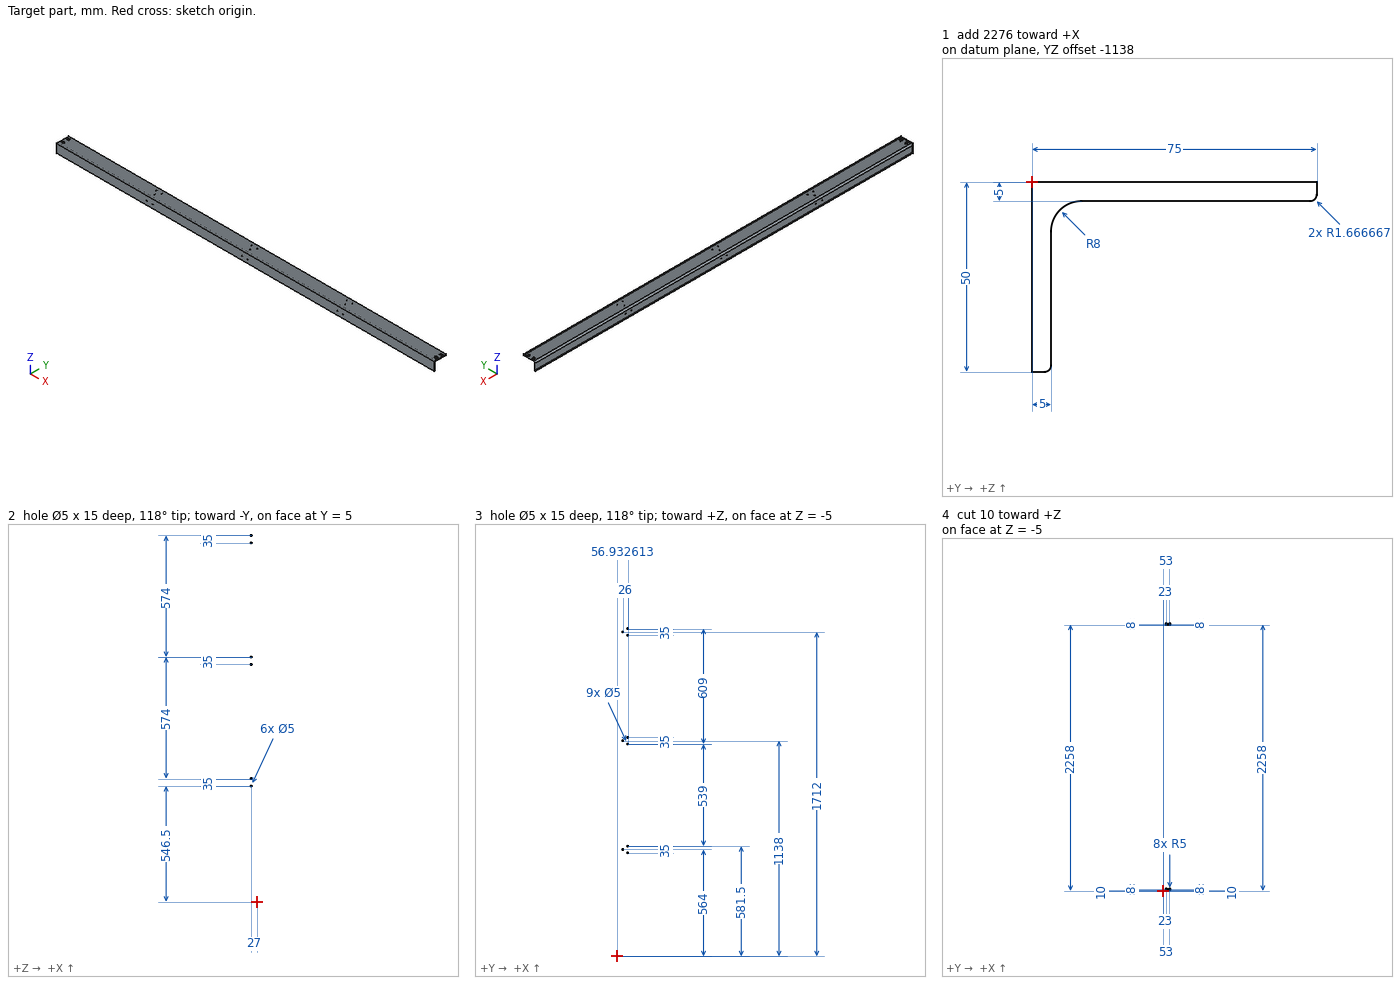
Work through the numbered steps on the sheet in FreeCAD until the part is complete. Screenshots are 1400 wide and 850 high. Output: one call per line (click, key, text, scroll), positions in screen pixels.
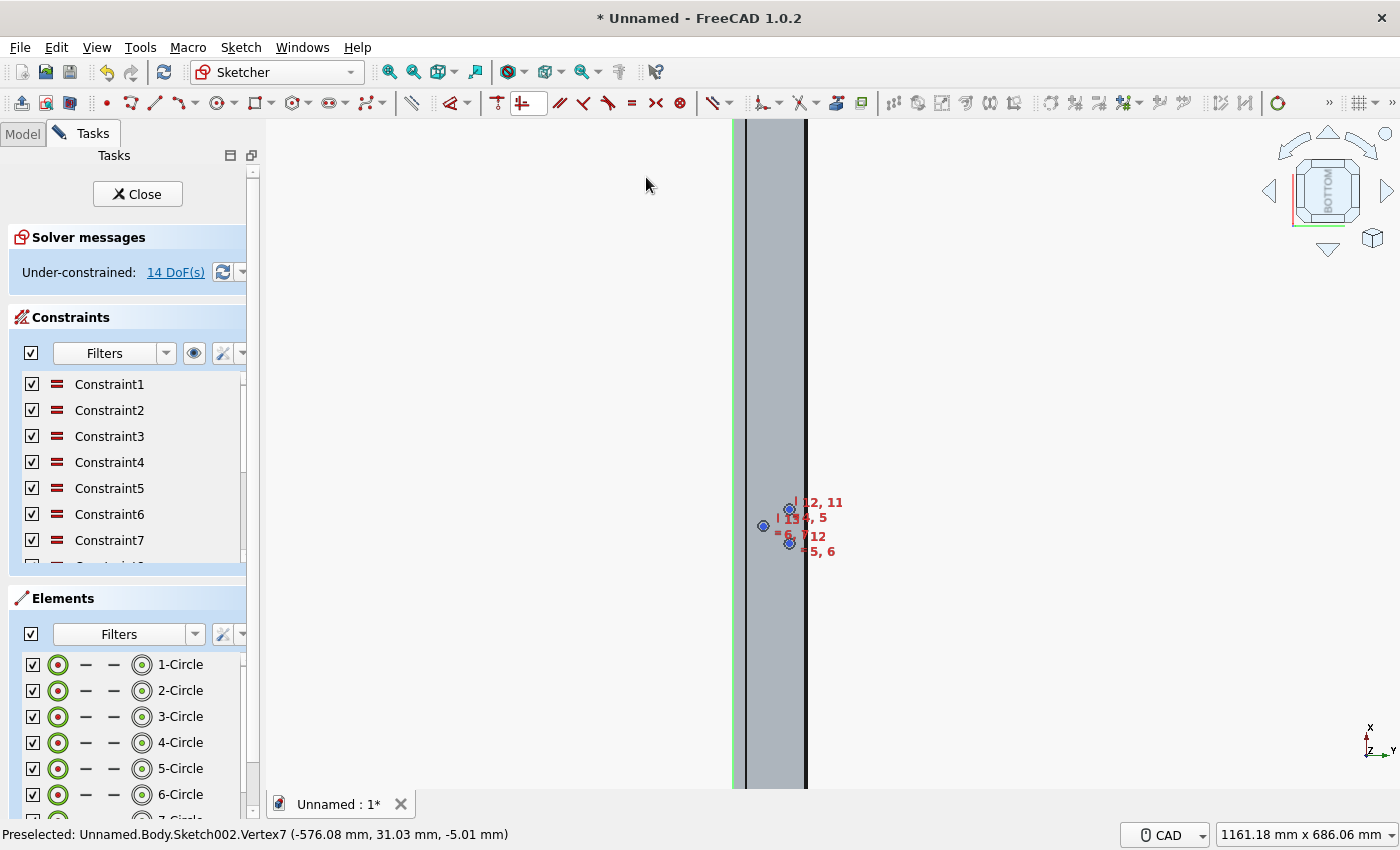
scroll(765, 528, down, 7)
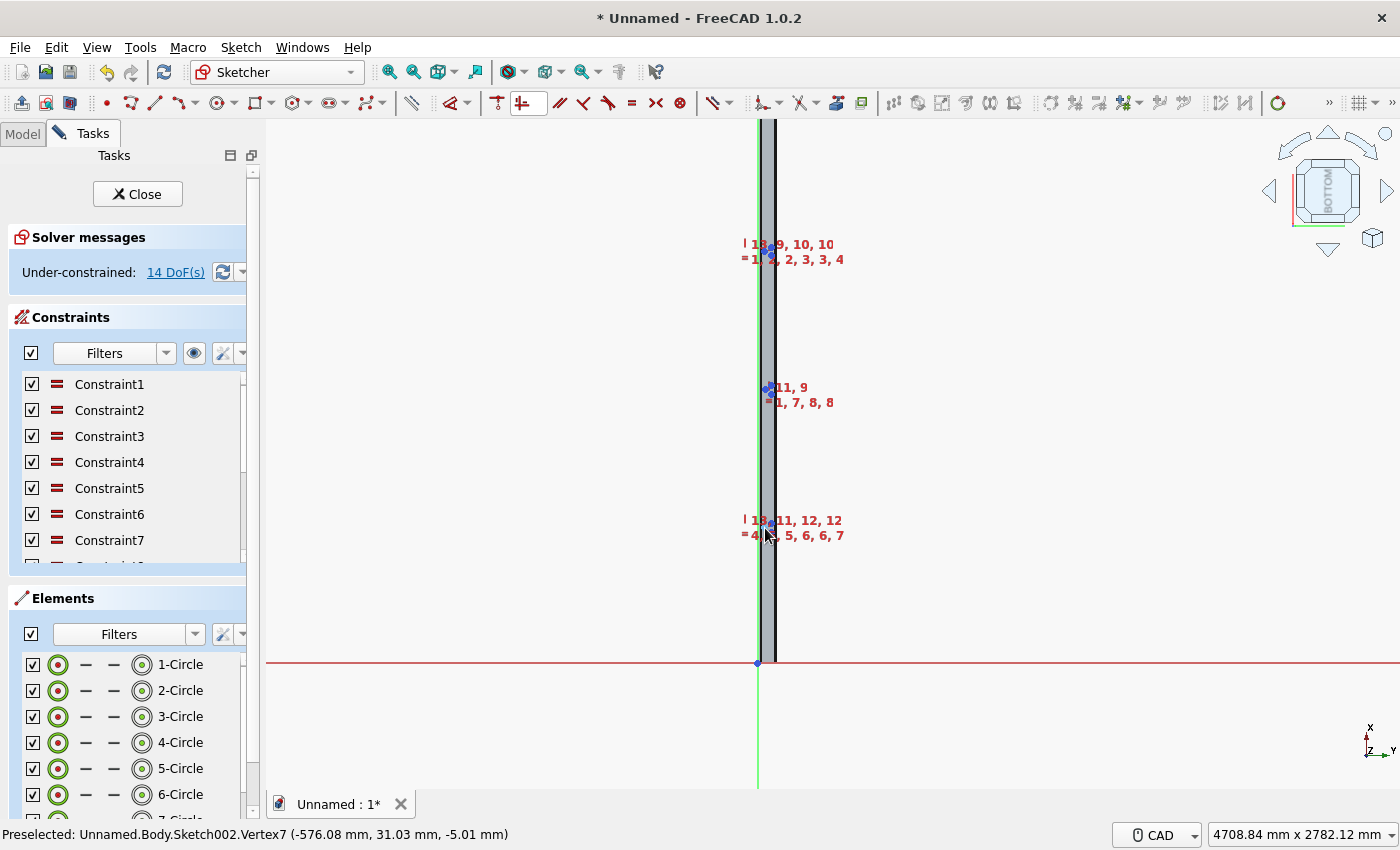
scroll(771, 394, up, 3)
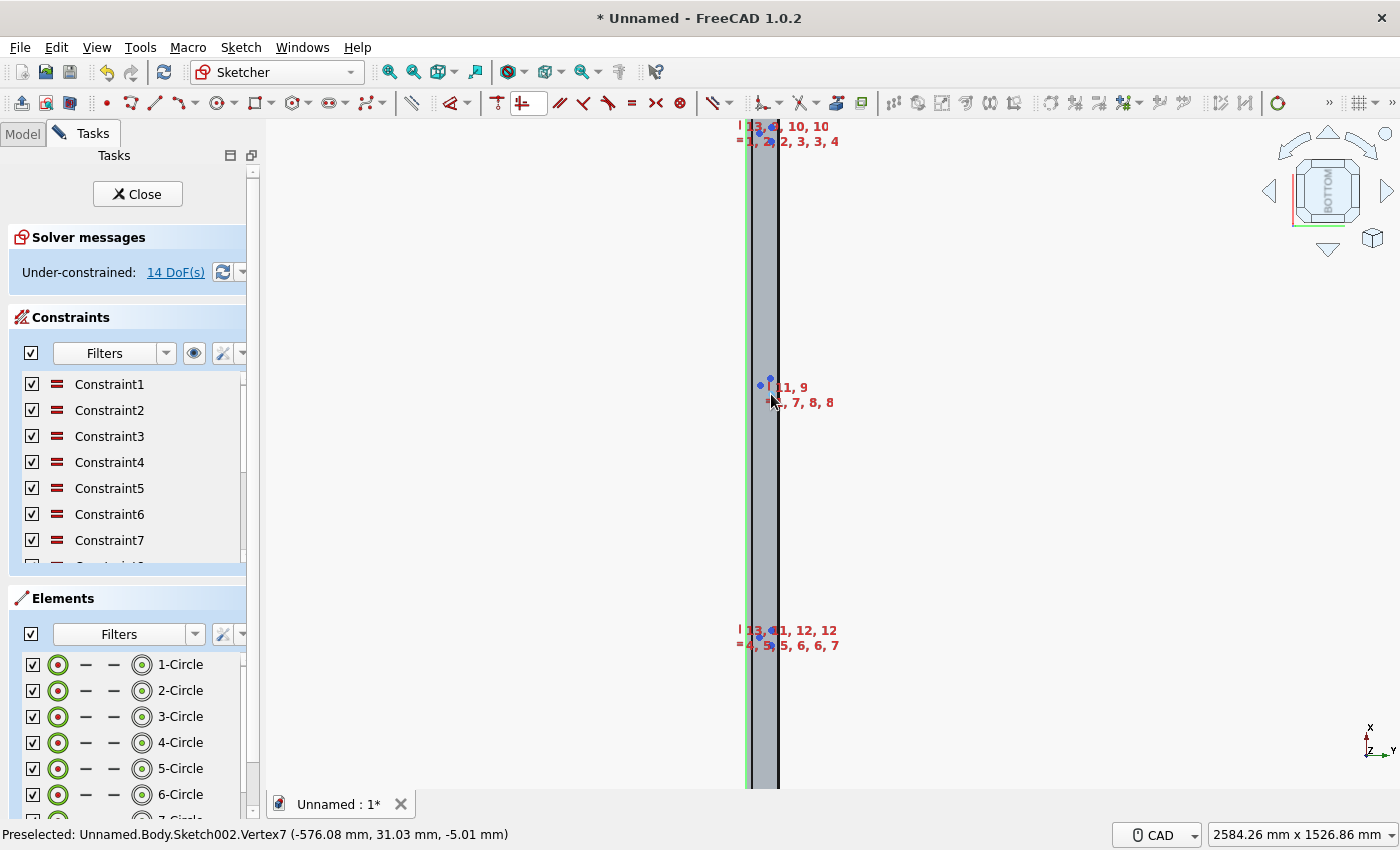
click(771, 394)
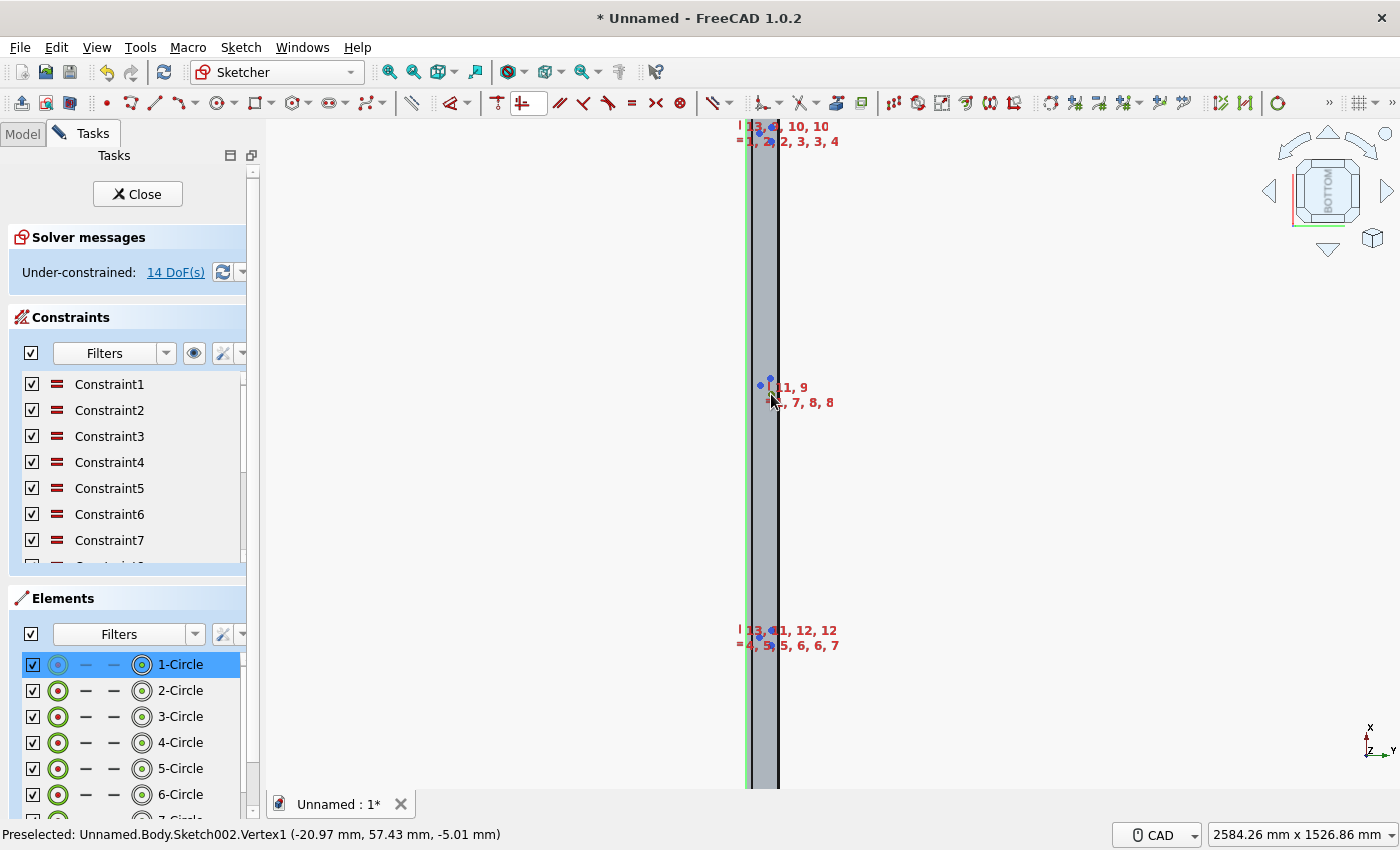
click(771, 378)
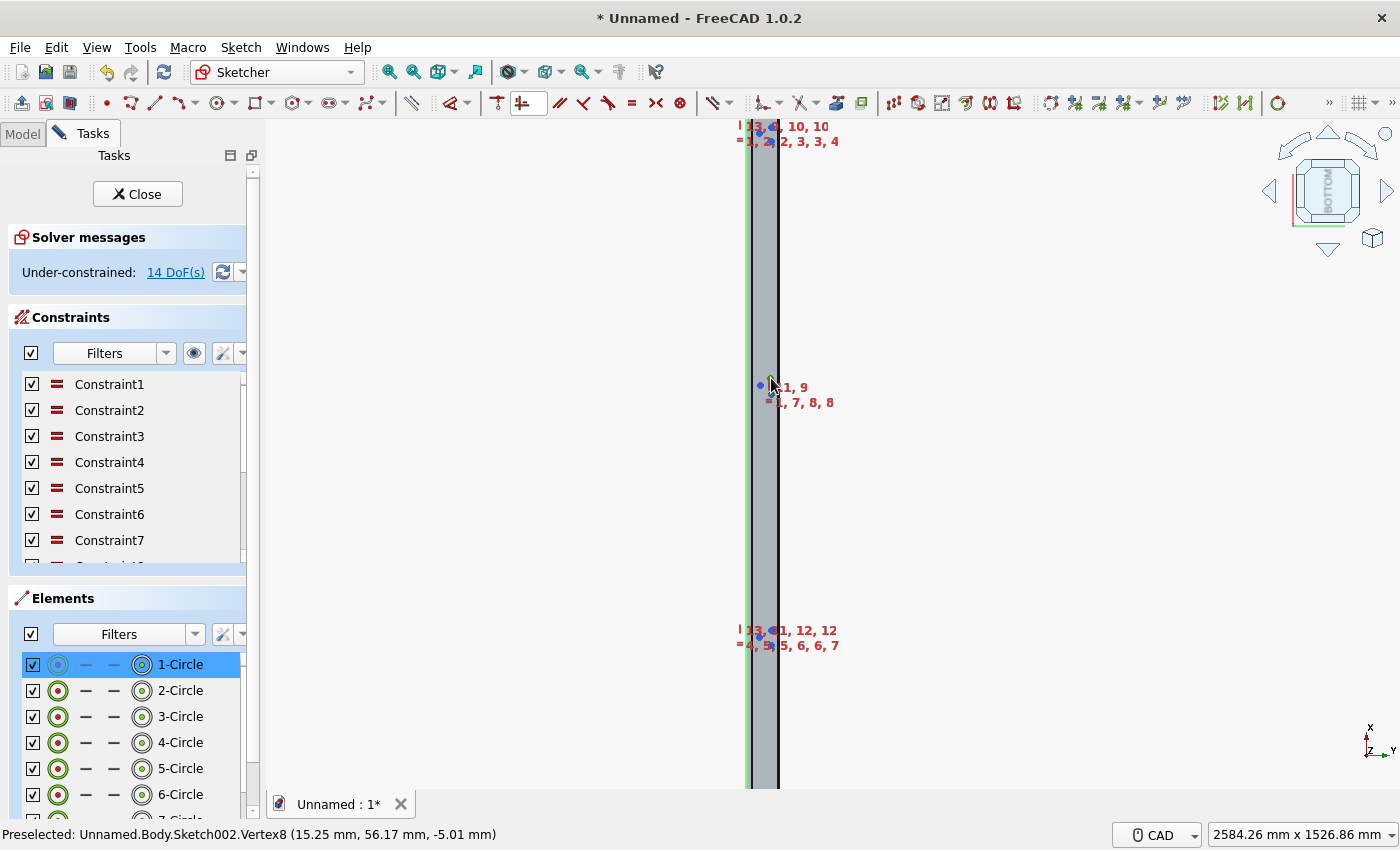
click(542, 104)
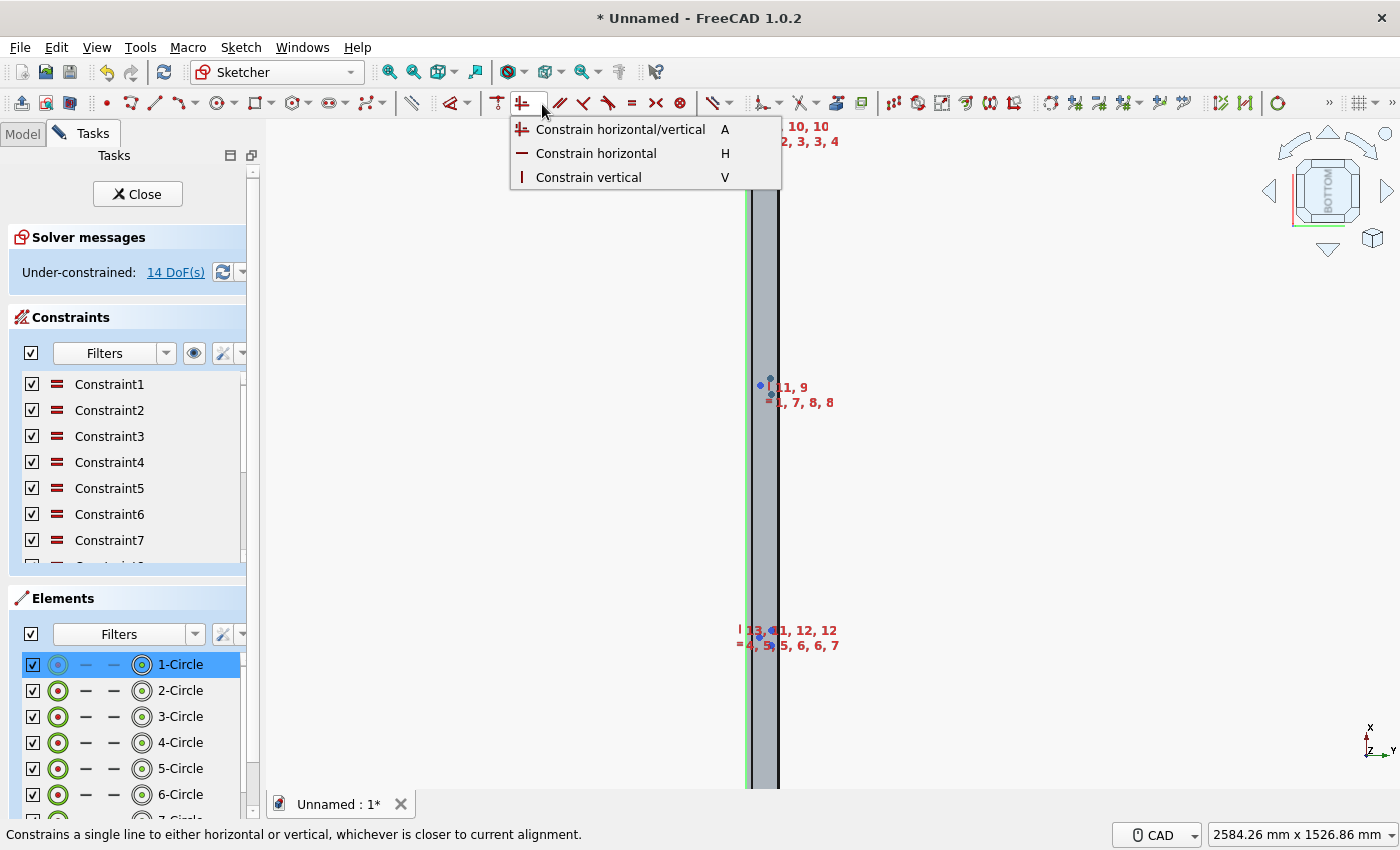
click(646, 177)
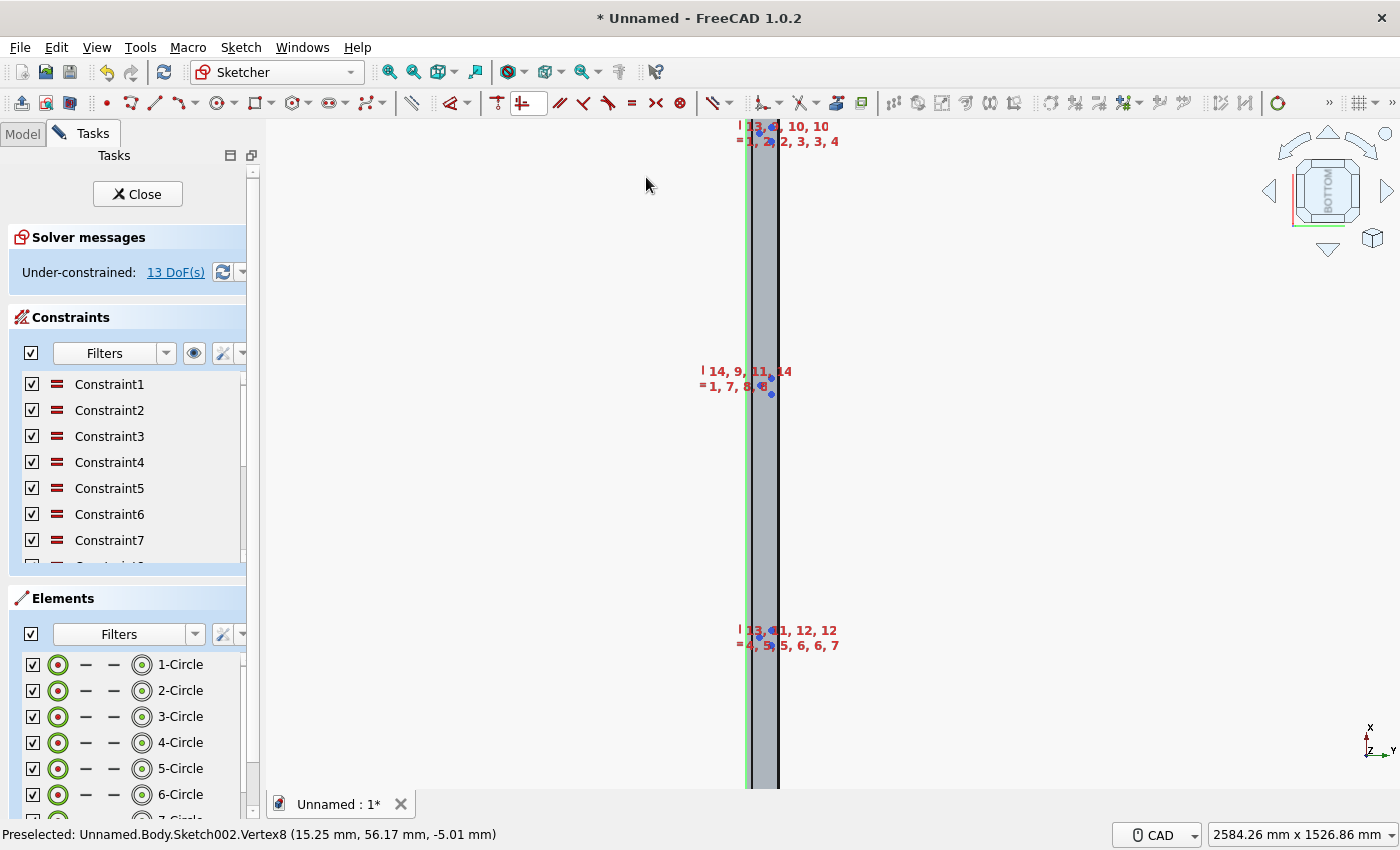
scroll(771, 393, down, 3)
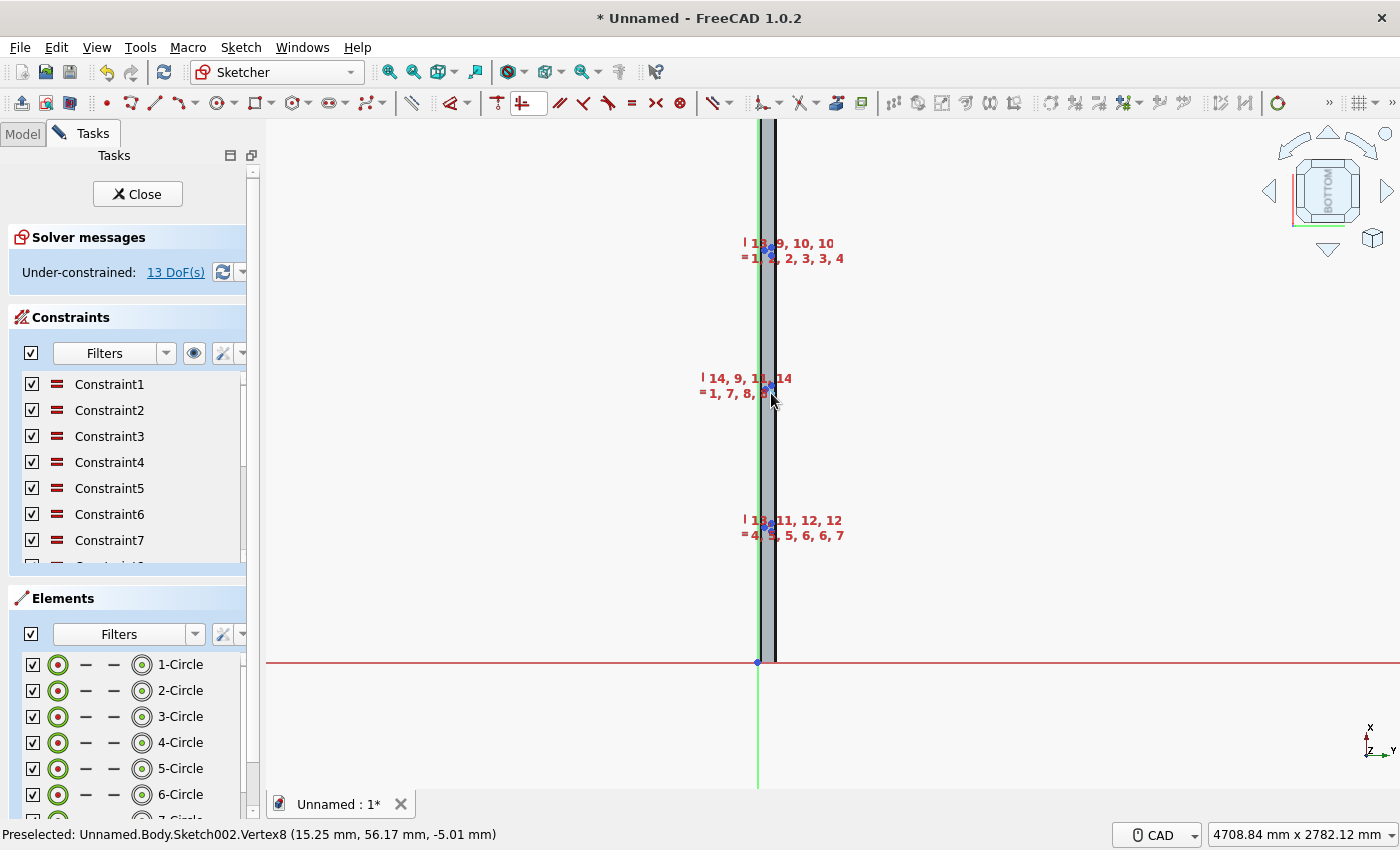
scroll(765, 251, up, 3)